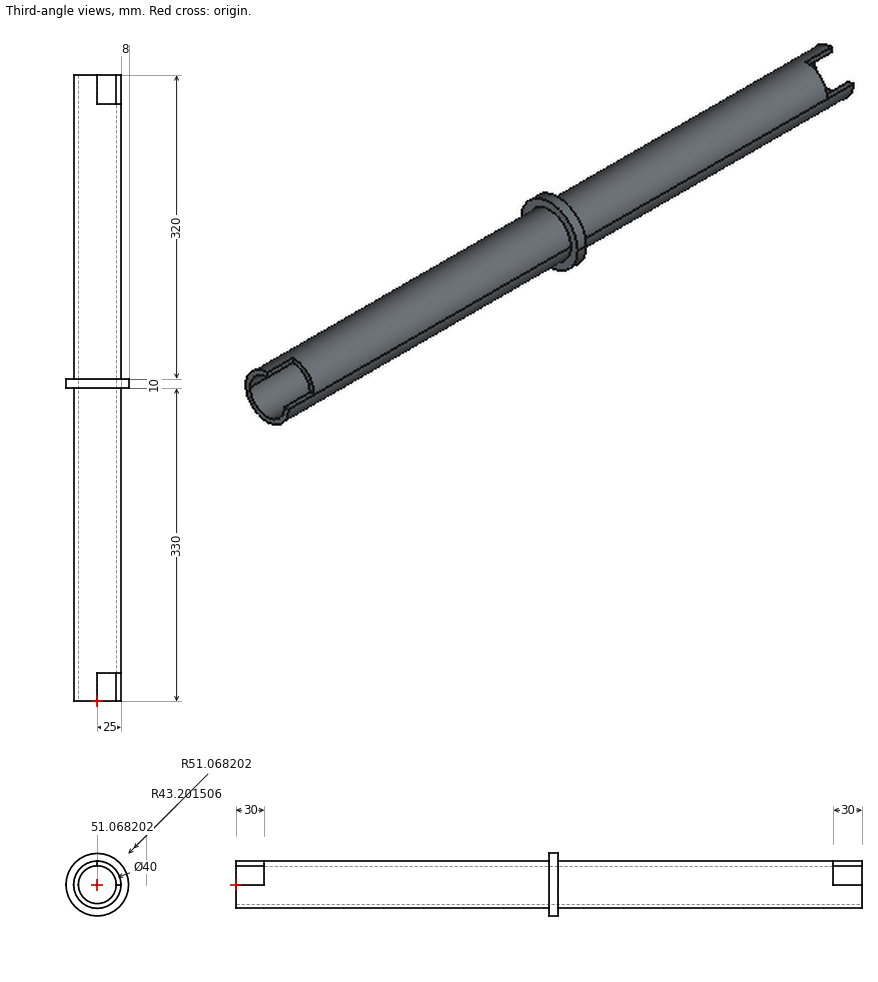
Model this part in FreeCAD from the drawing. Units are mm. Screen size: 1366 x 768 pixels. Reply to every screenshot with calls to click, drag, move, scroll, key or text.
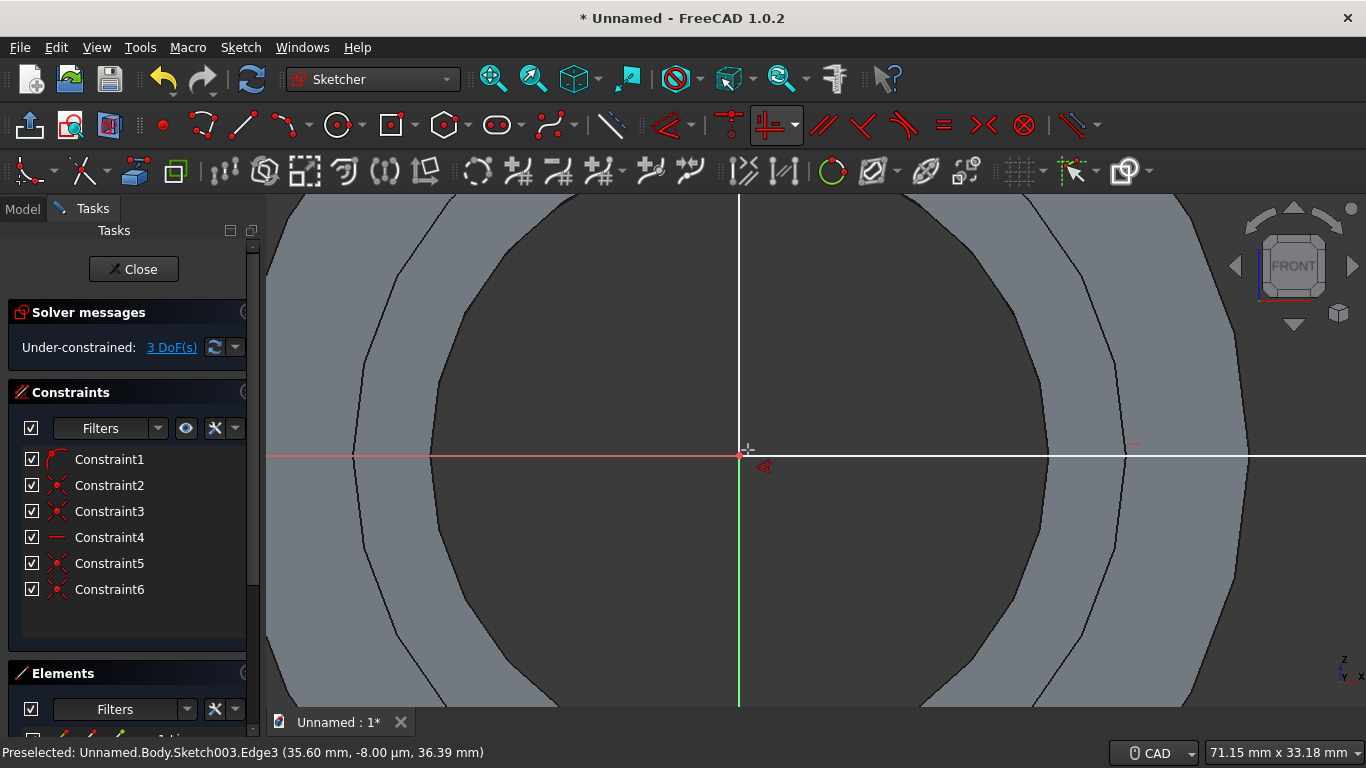
scroll(522, 677, down, 5)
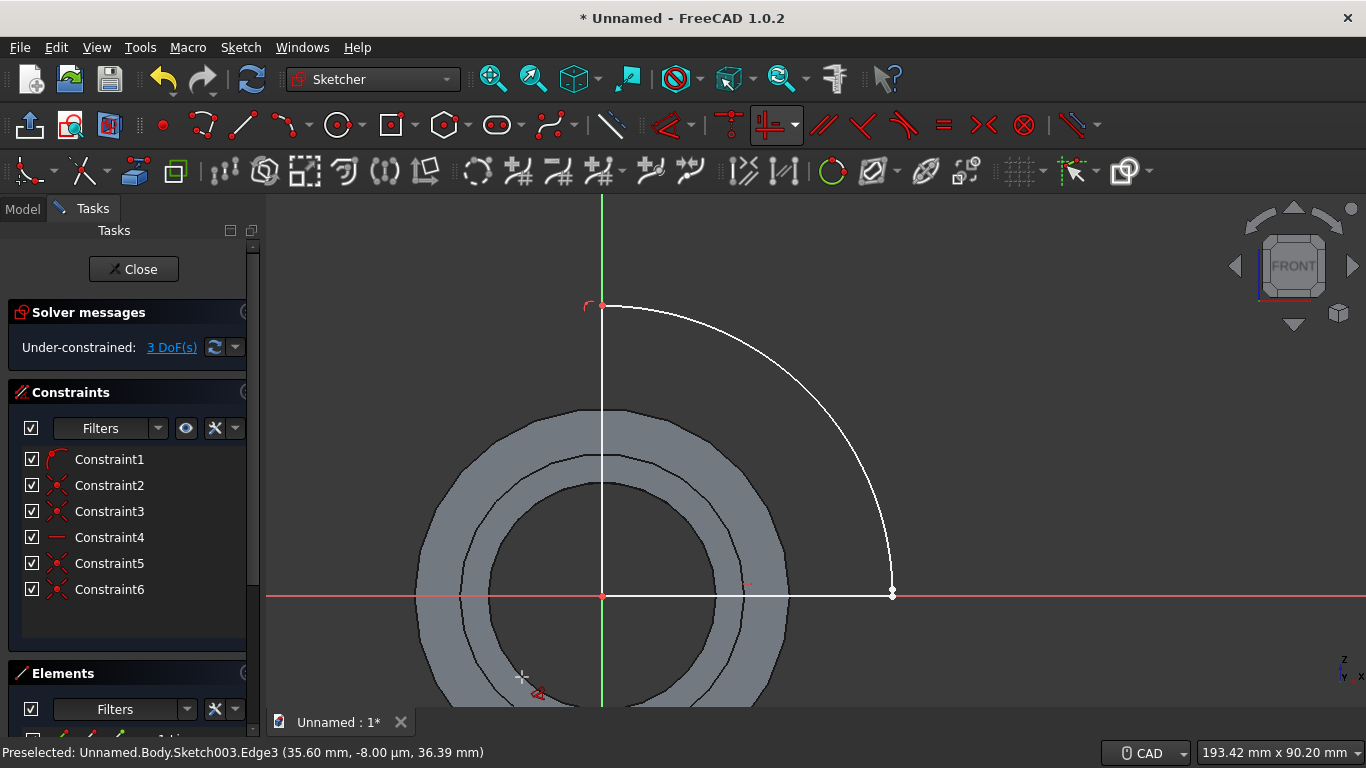
click(859, 460)
click(887, 445)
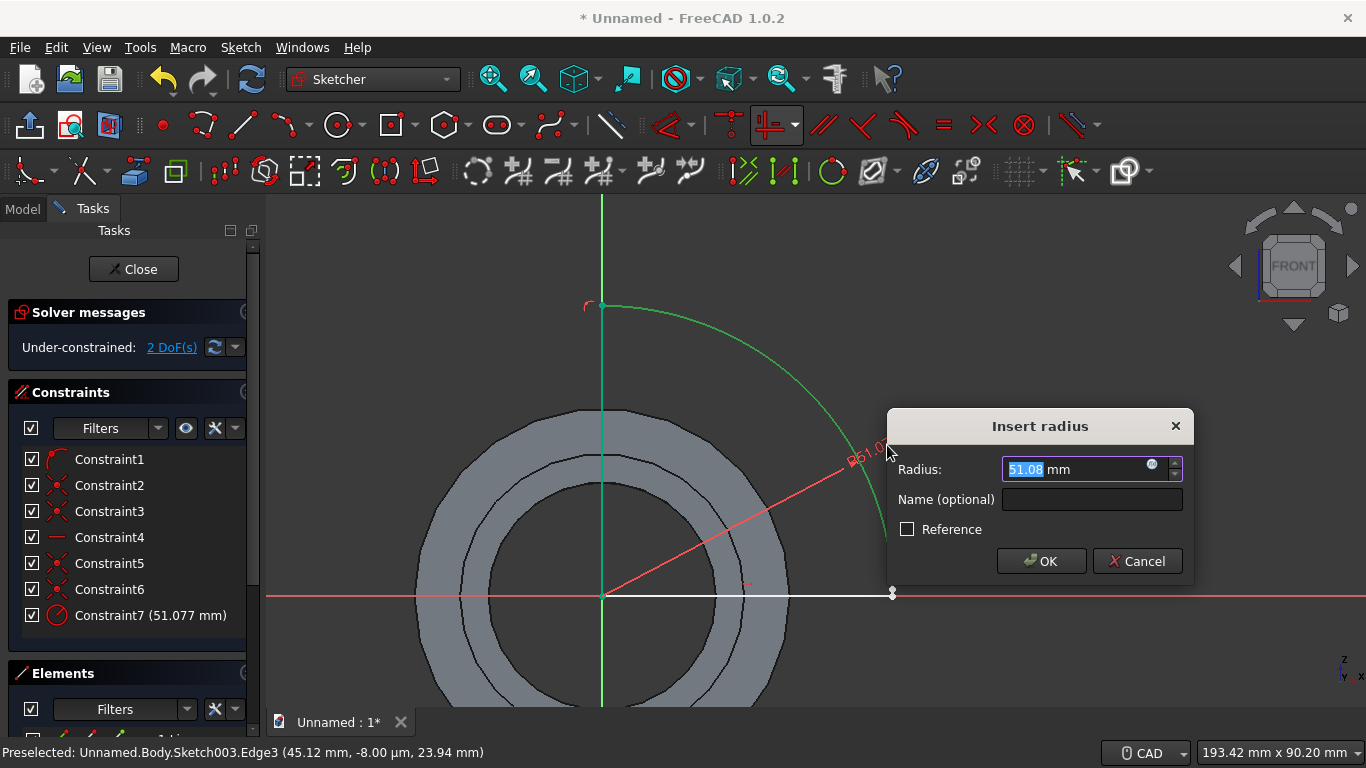
text(51.068202)
key(Return)
key(Escape)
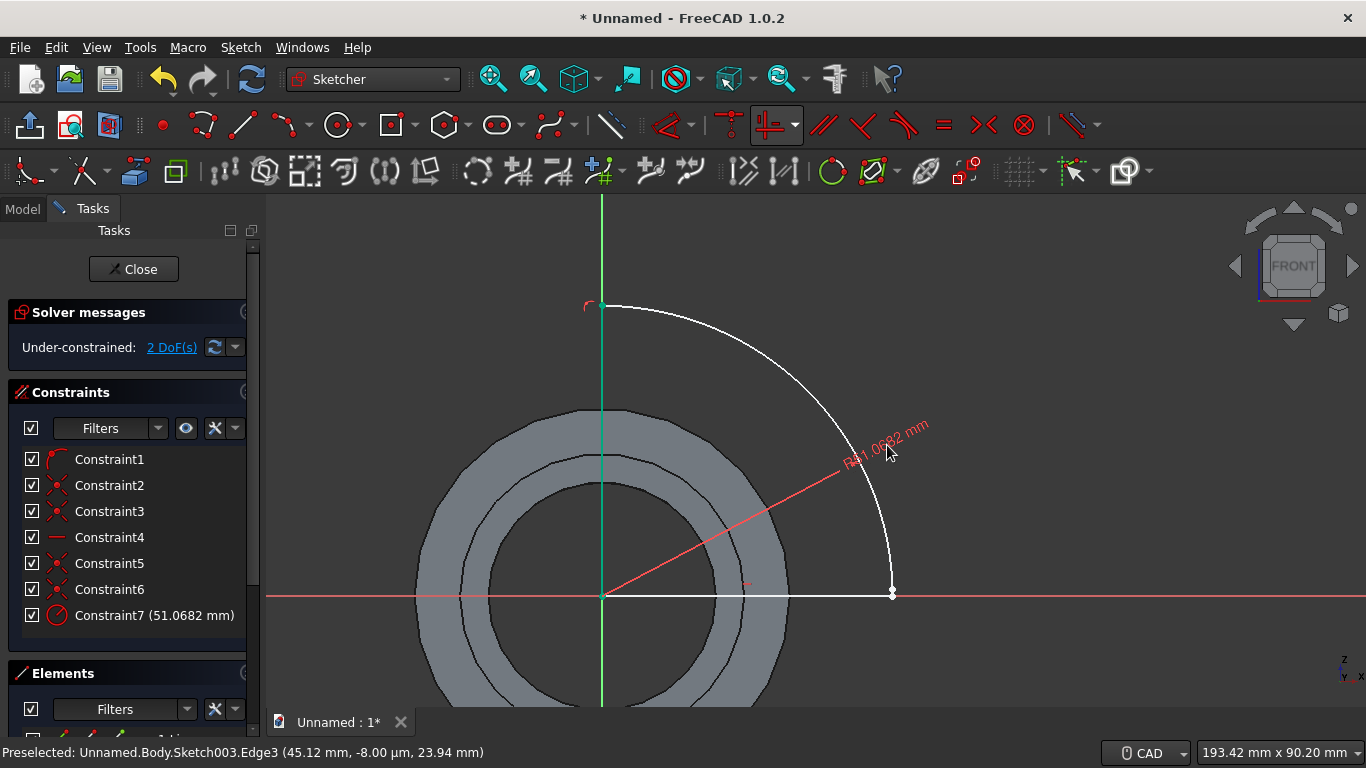
click(892, 589)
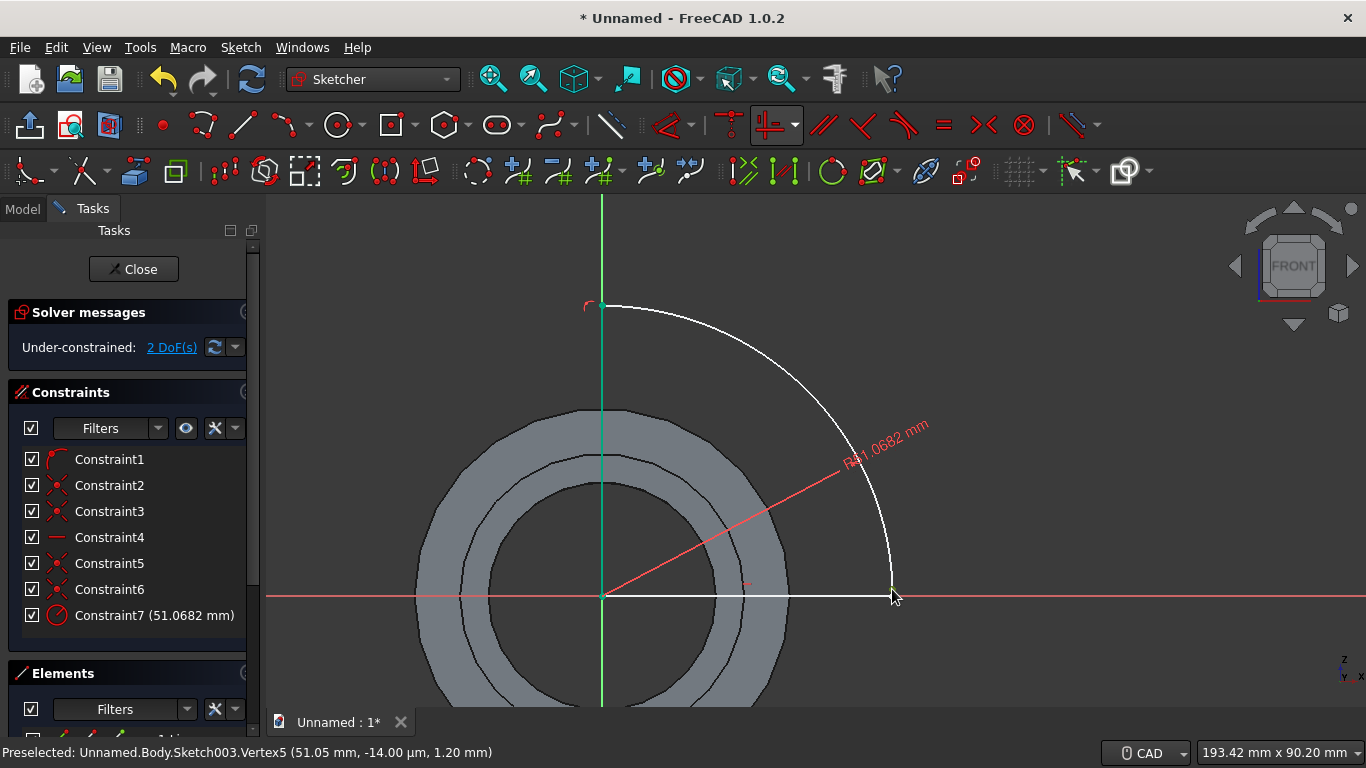
click(359, 596)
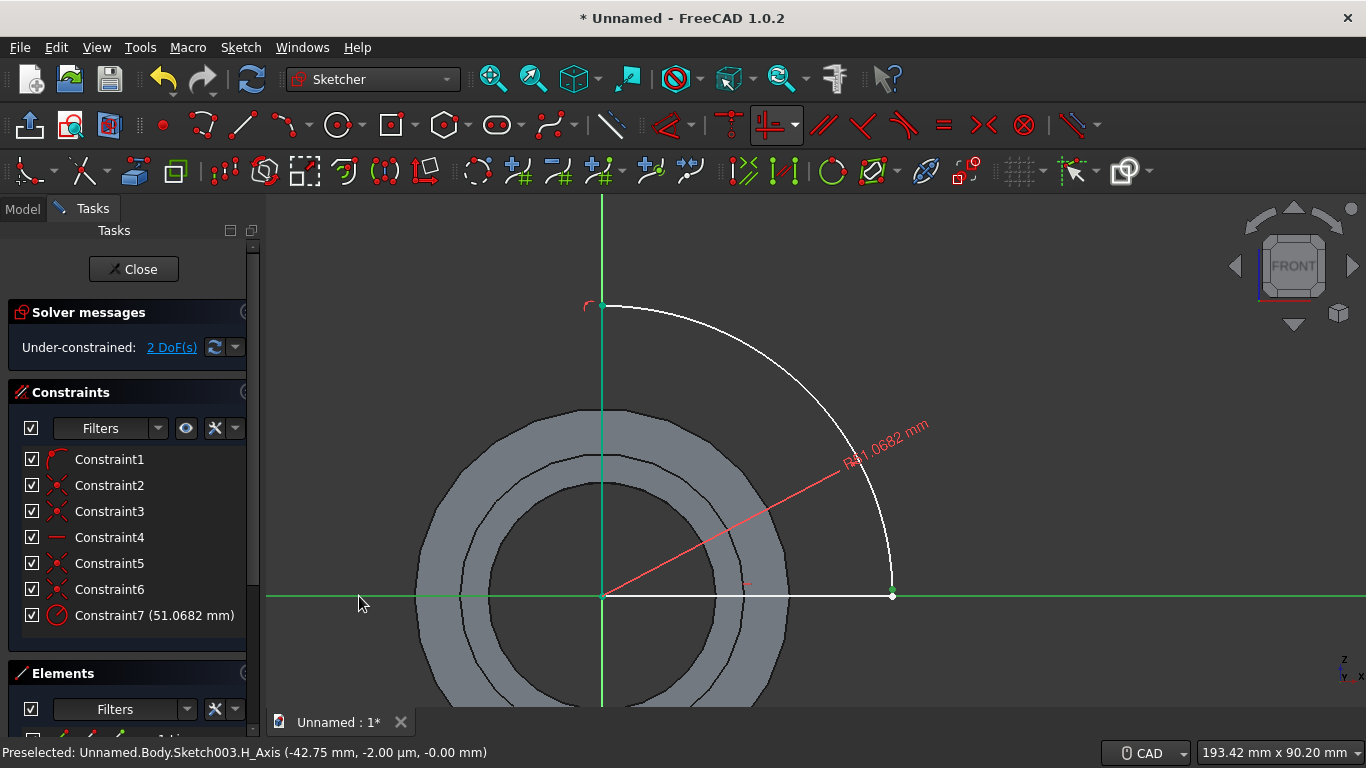
click(730, 126)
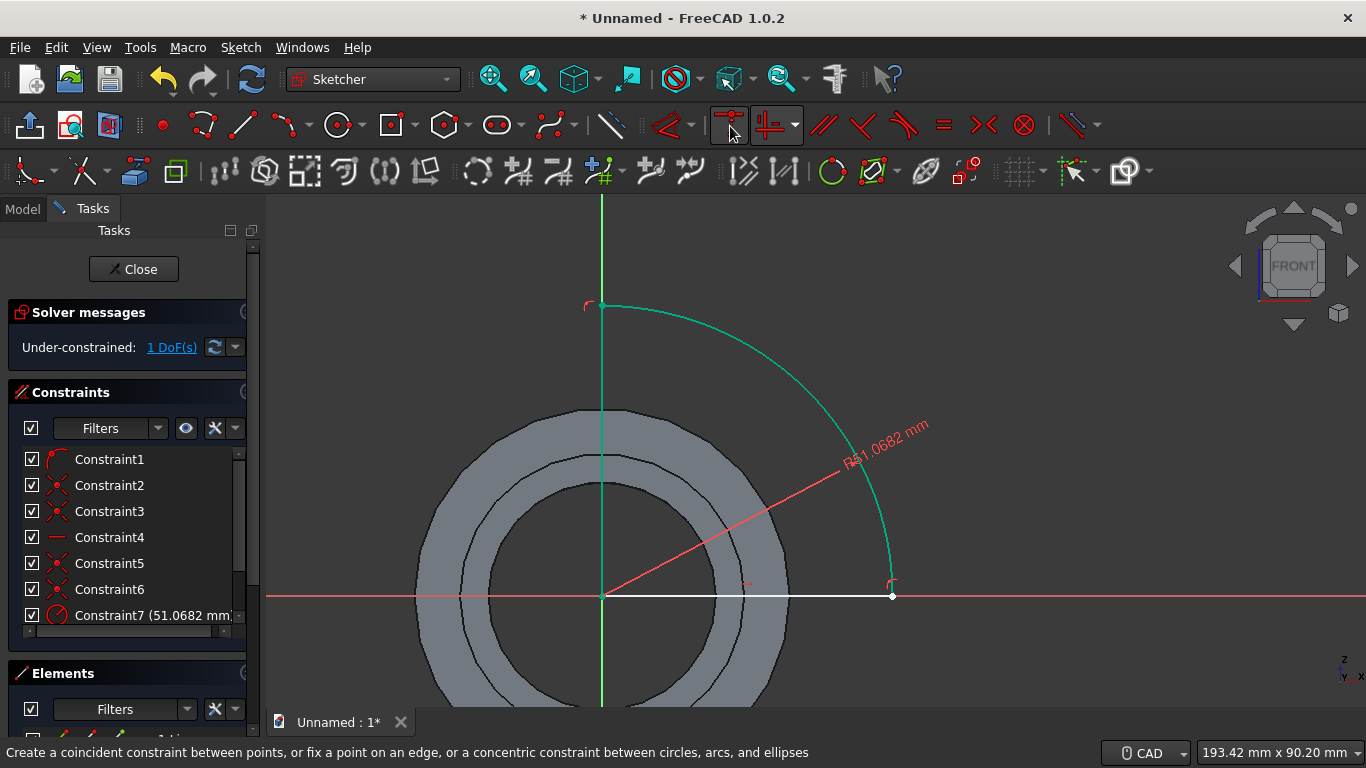
click(666, 126)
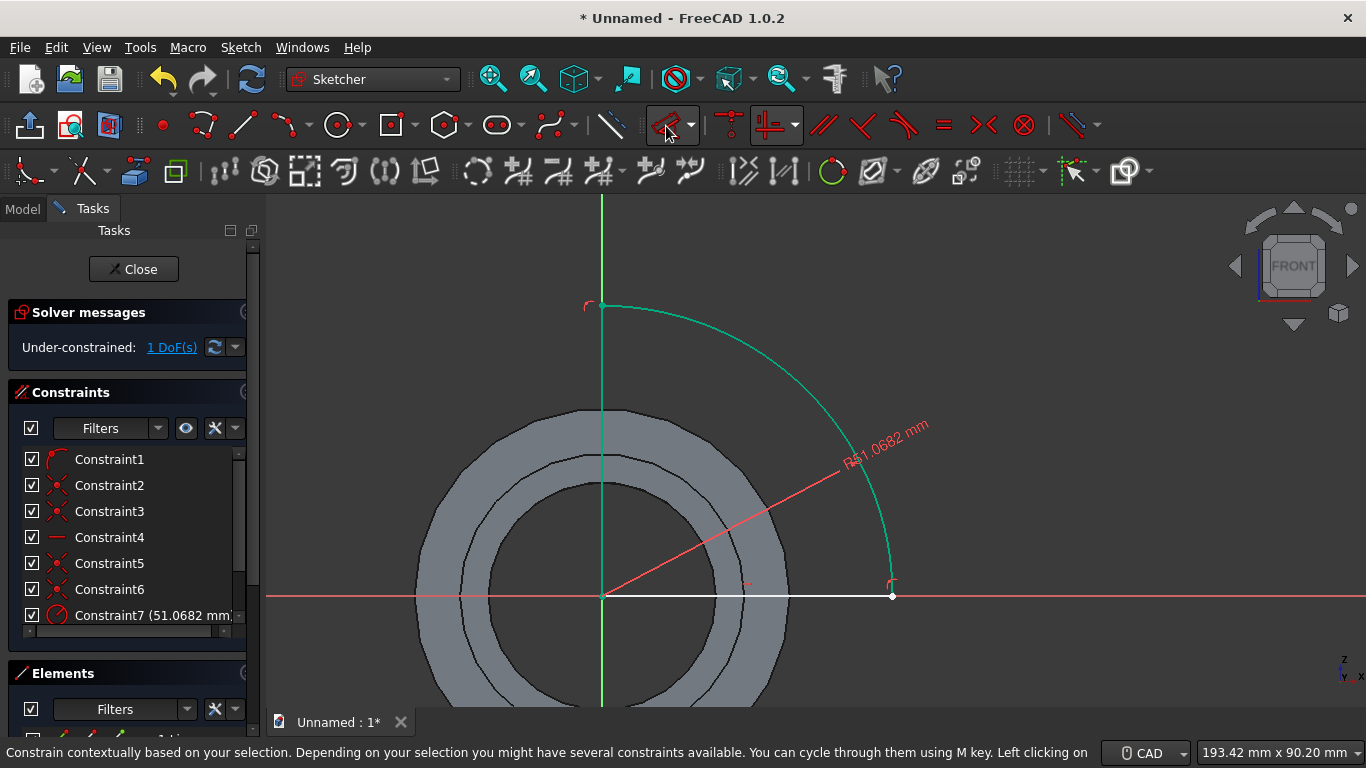
click(689, 596)
click(747, 630)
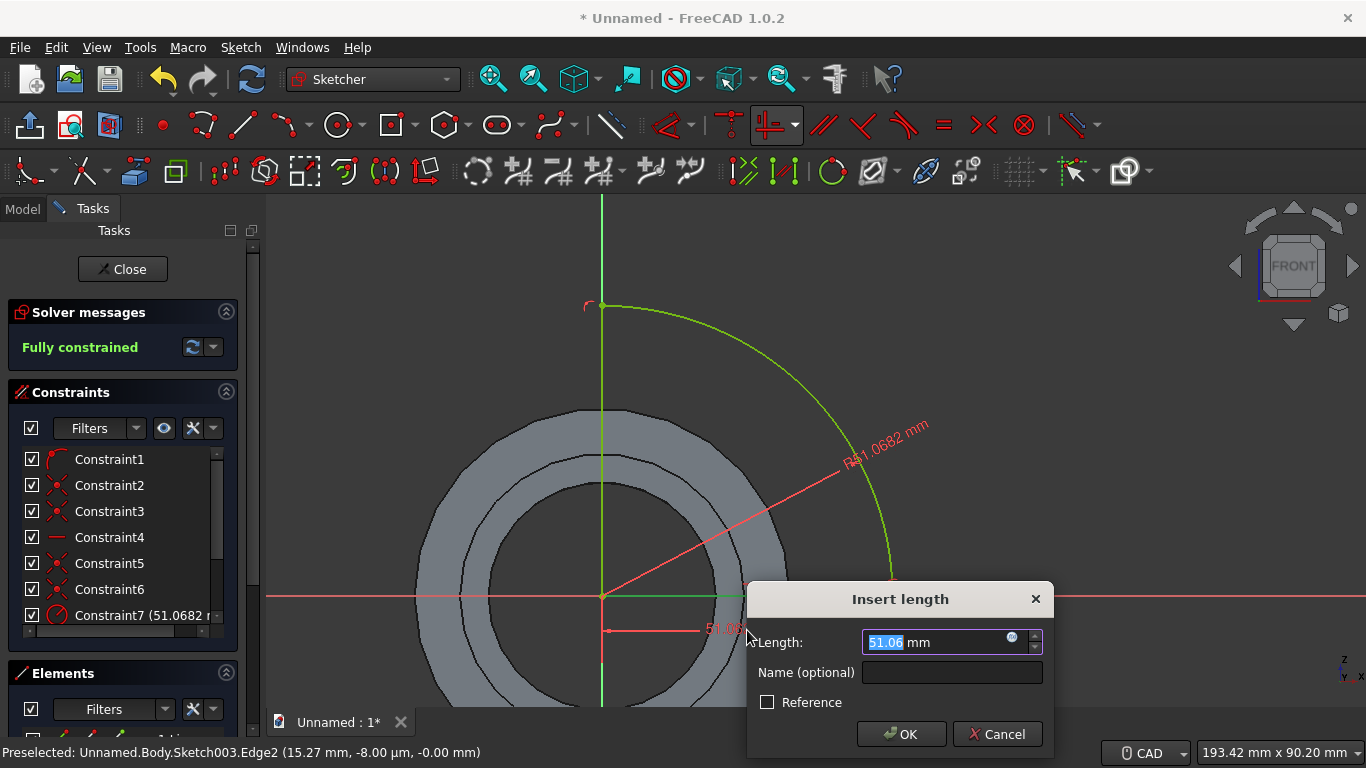
text(51.068202)
key(Return)
key(Escape)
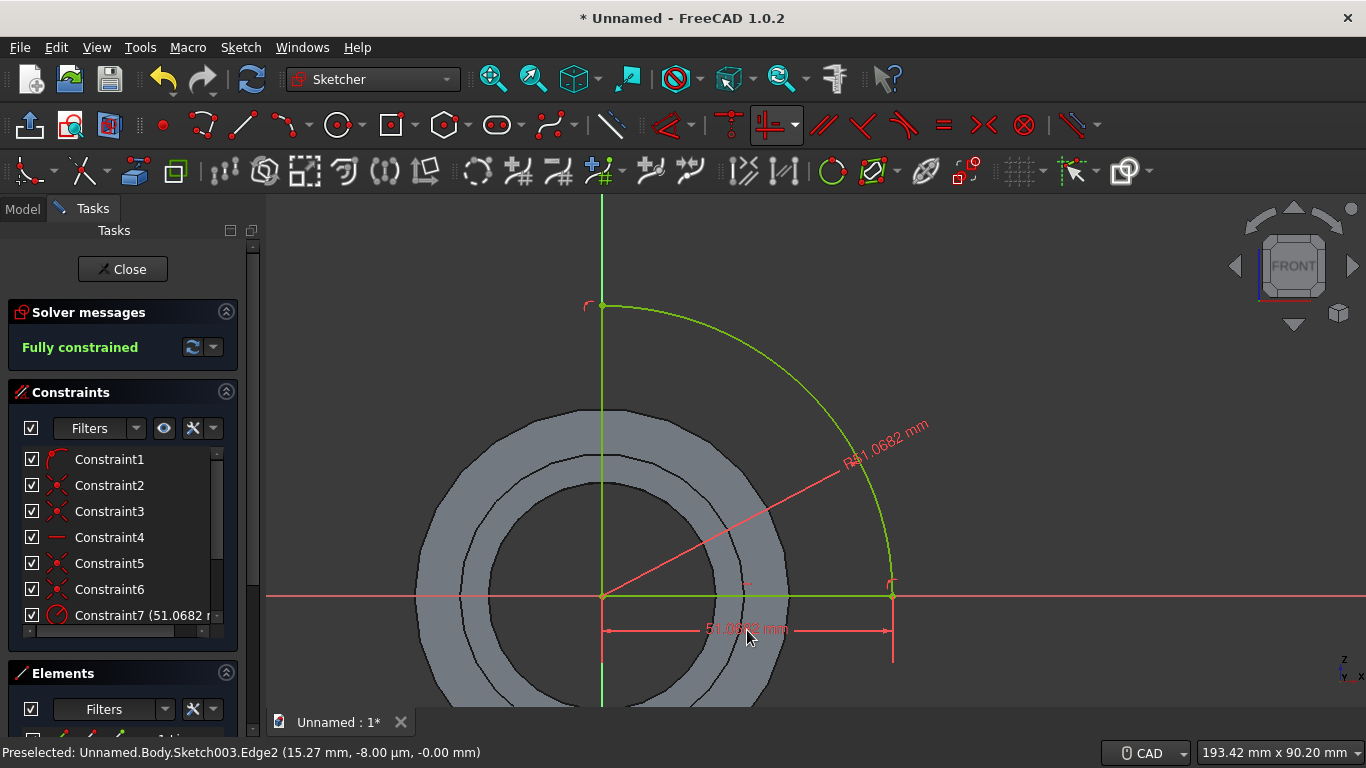
click(123, 269)